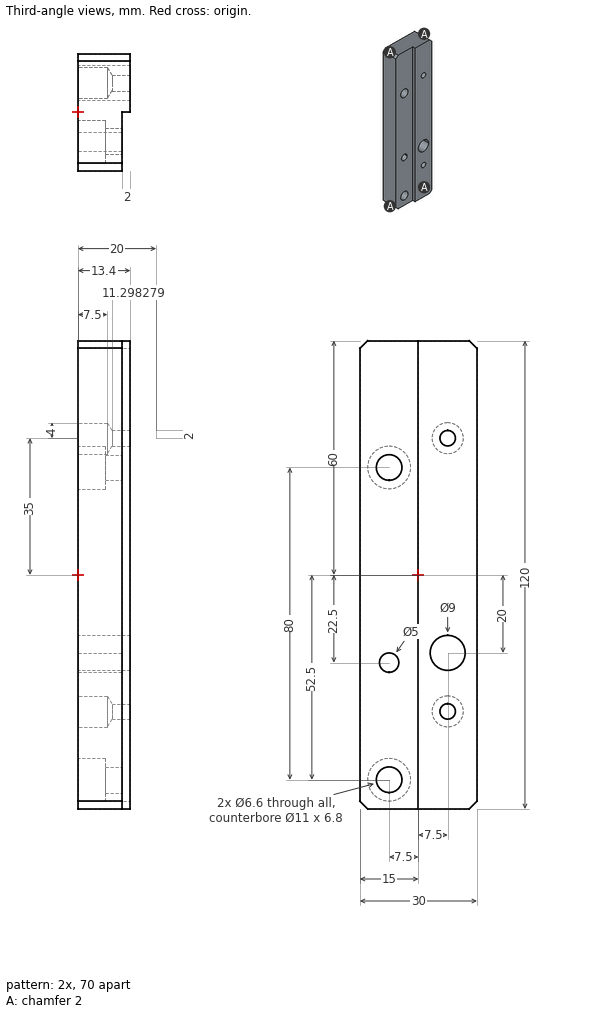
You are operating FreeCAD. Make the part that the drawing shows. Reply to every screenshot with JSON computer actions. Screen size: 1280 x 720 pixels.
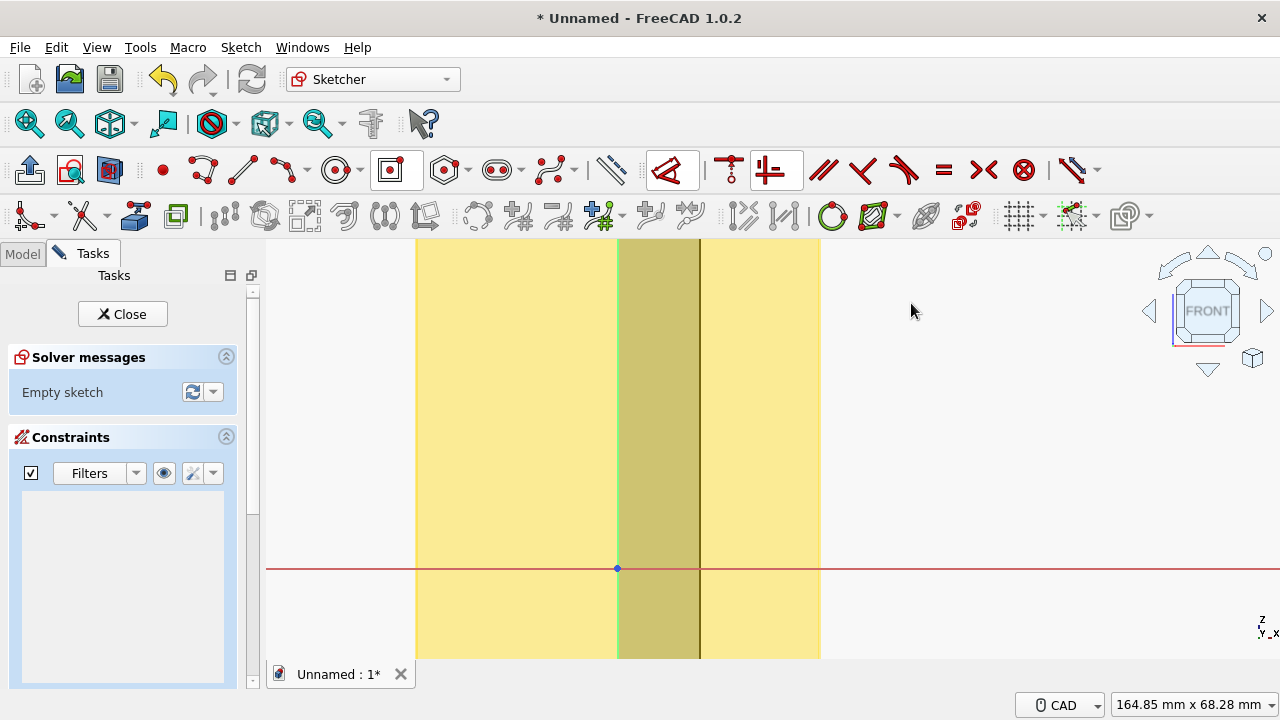
{"action": "left_click", "coordinate": [204, 170]}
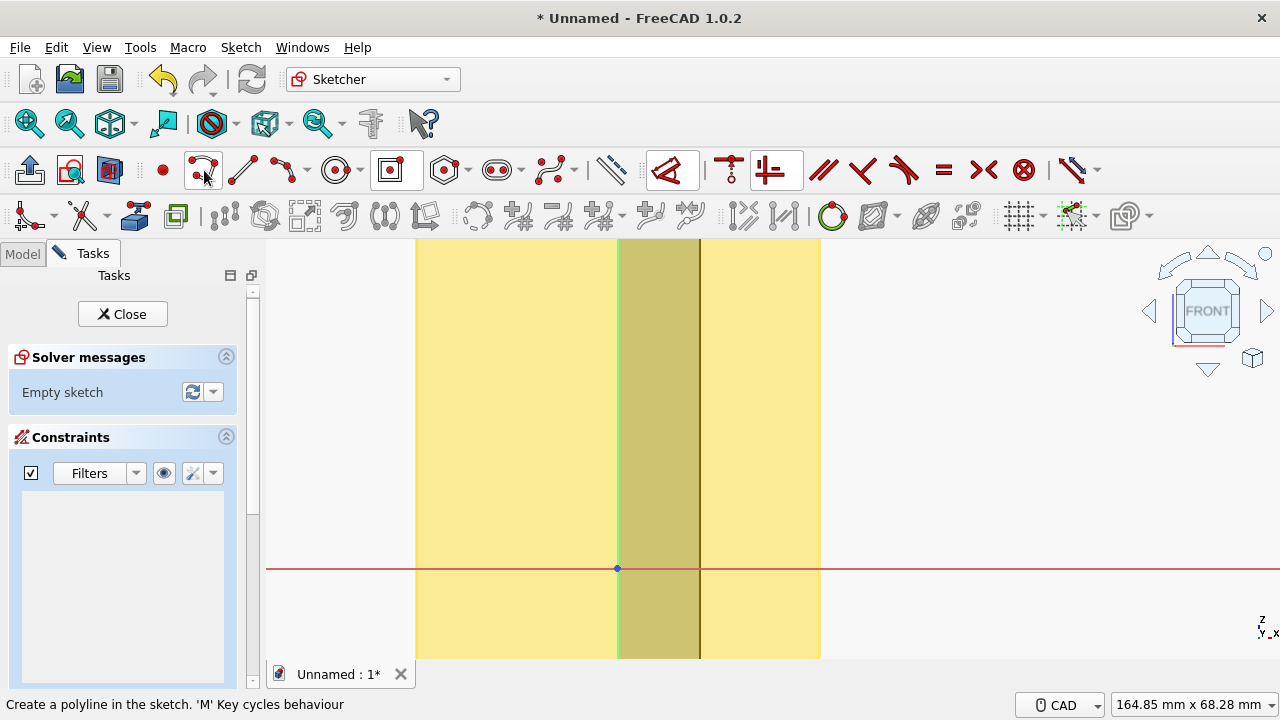
{"action": "left_click", "coordinate": [618, 354]}
{"action": "left_click", "coordinate": [627, 329]}
{"action": "left_click", "coordinate": [664, 329]}
{"action": "left_click", "coordinate": [671, 341]}
{"action": "left_click", "coordinate": [741, 341]}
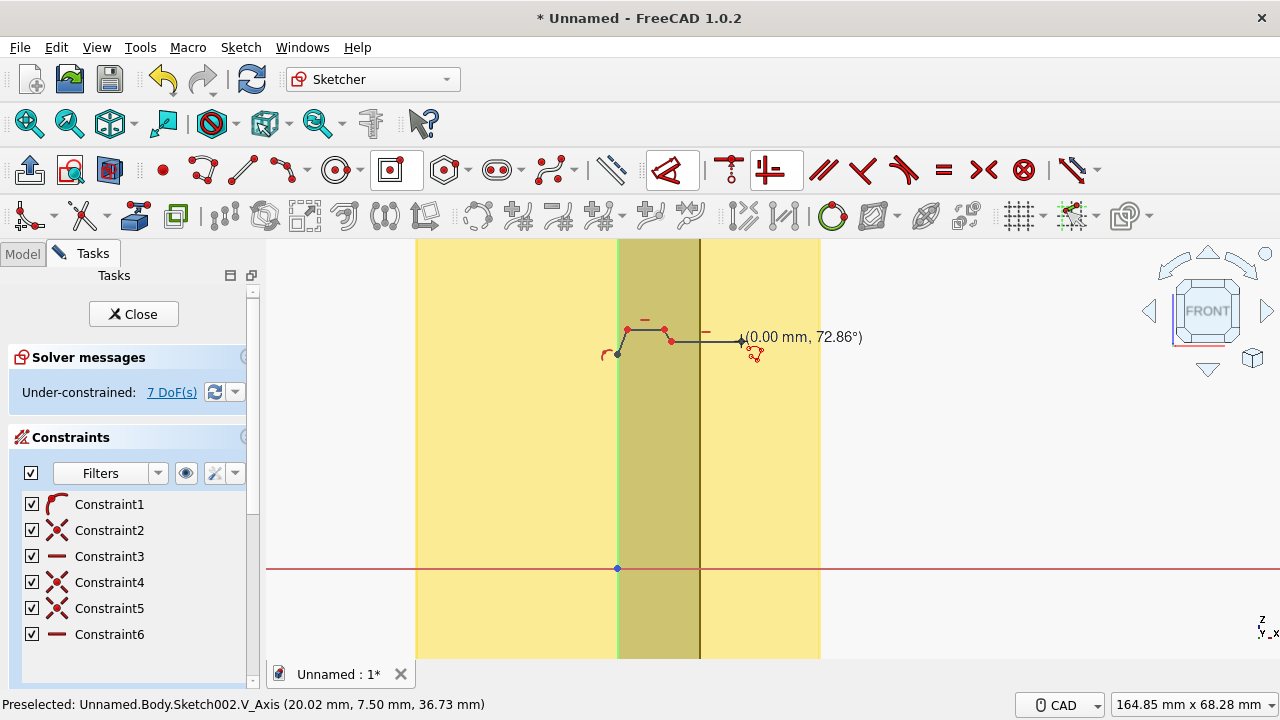
{"action": "scroll", "coordinate": [741, 354], "scroll_direction": "up", "scroll_amount": 2}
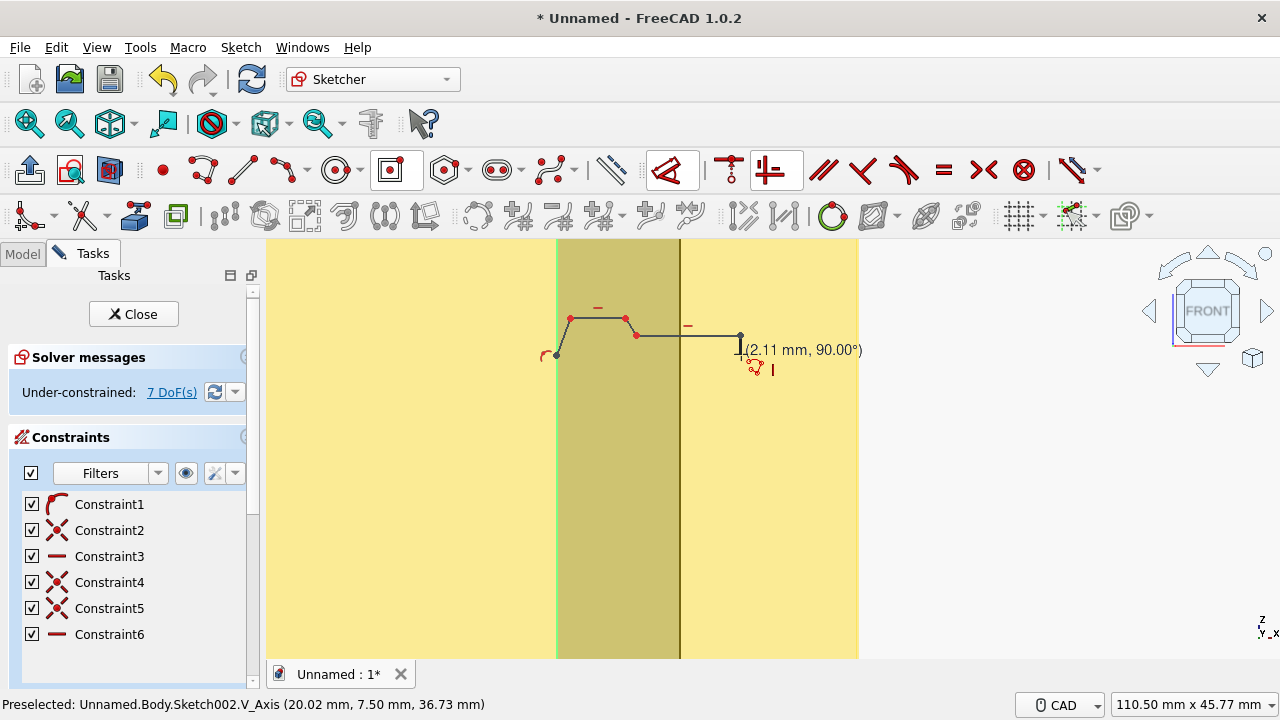
{"action": "left_click", "coordinate": [741, 353]}
{"action": "left_click", "coordinate": [557, 355]}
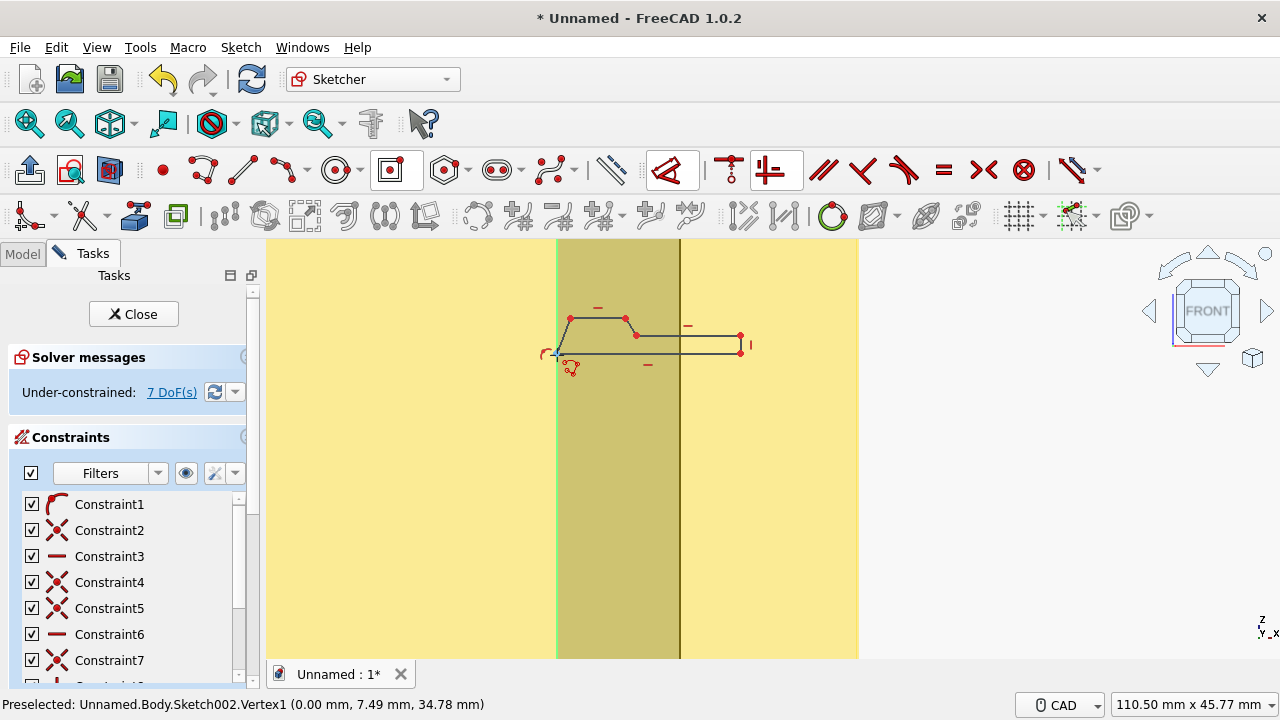
{"action": "left_click", "coordinate": [244, 170]}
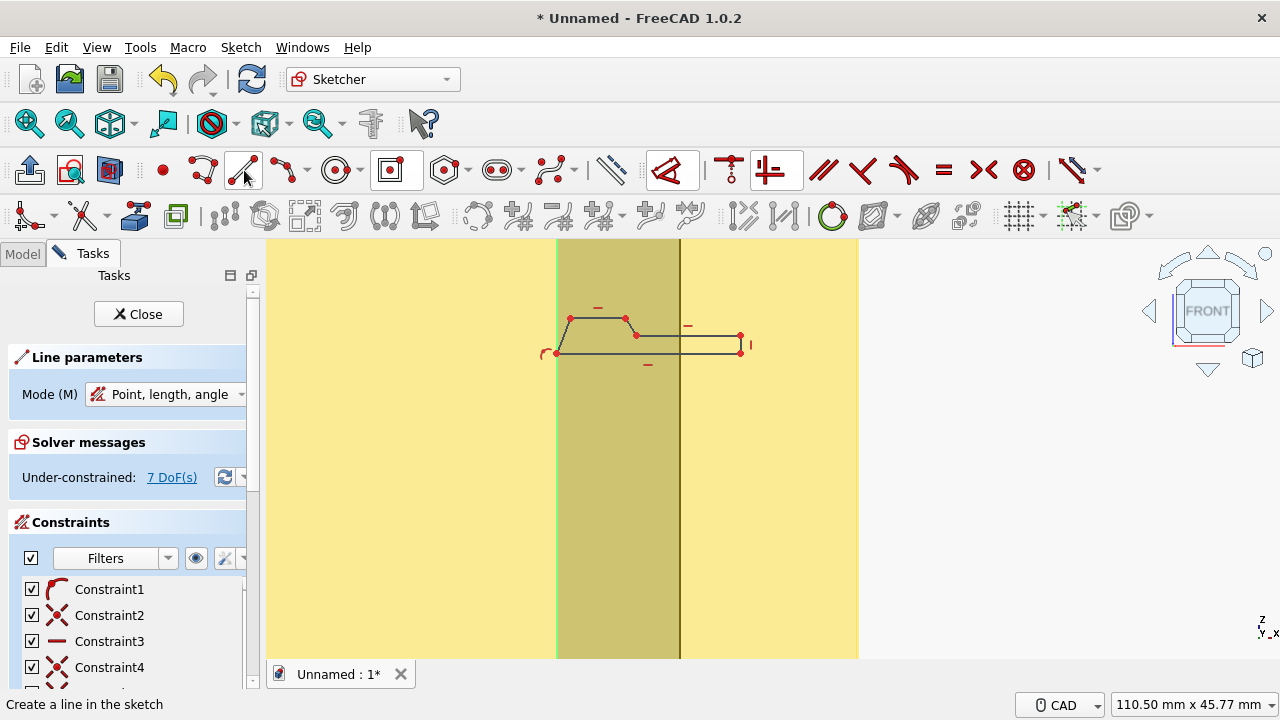
{"action": "left_click", "coordinate": [759, 353]}
{"action": "left_click", "coordinate": [814, 353]}
{"action": "key", "text": "Escape"}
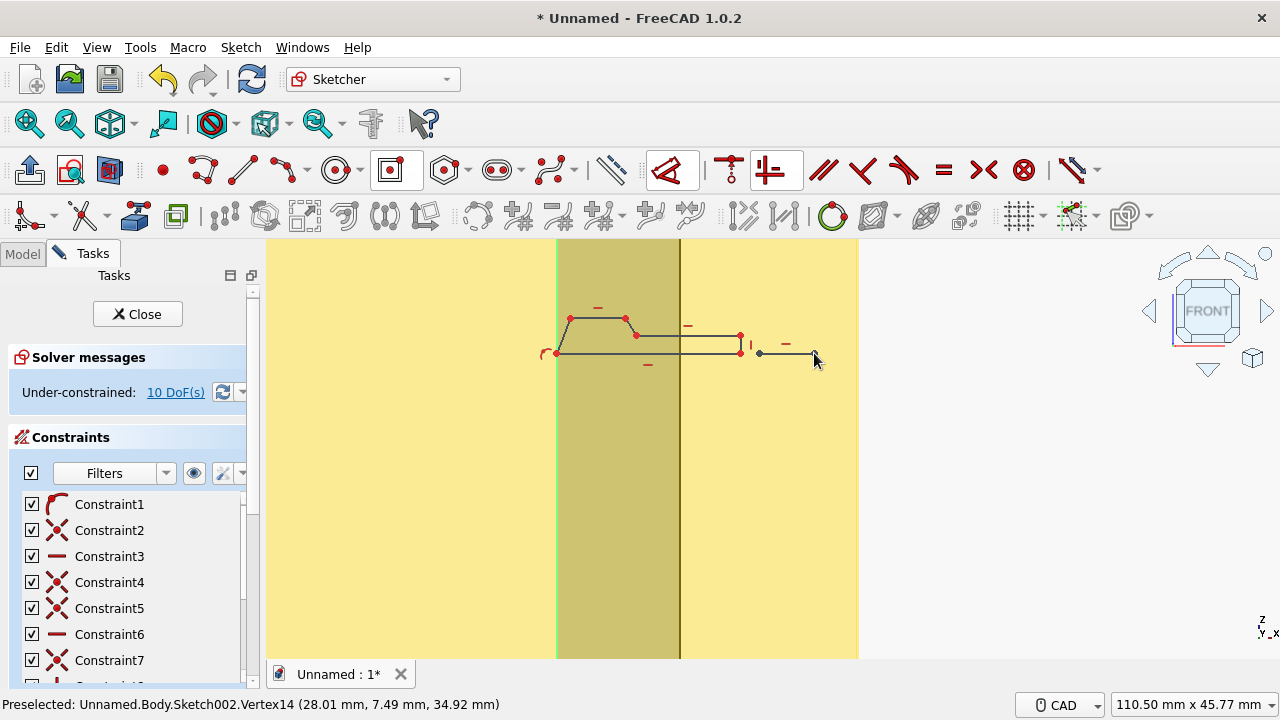
{"action": "left_click", "coordinate": [776, 354]}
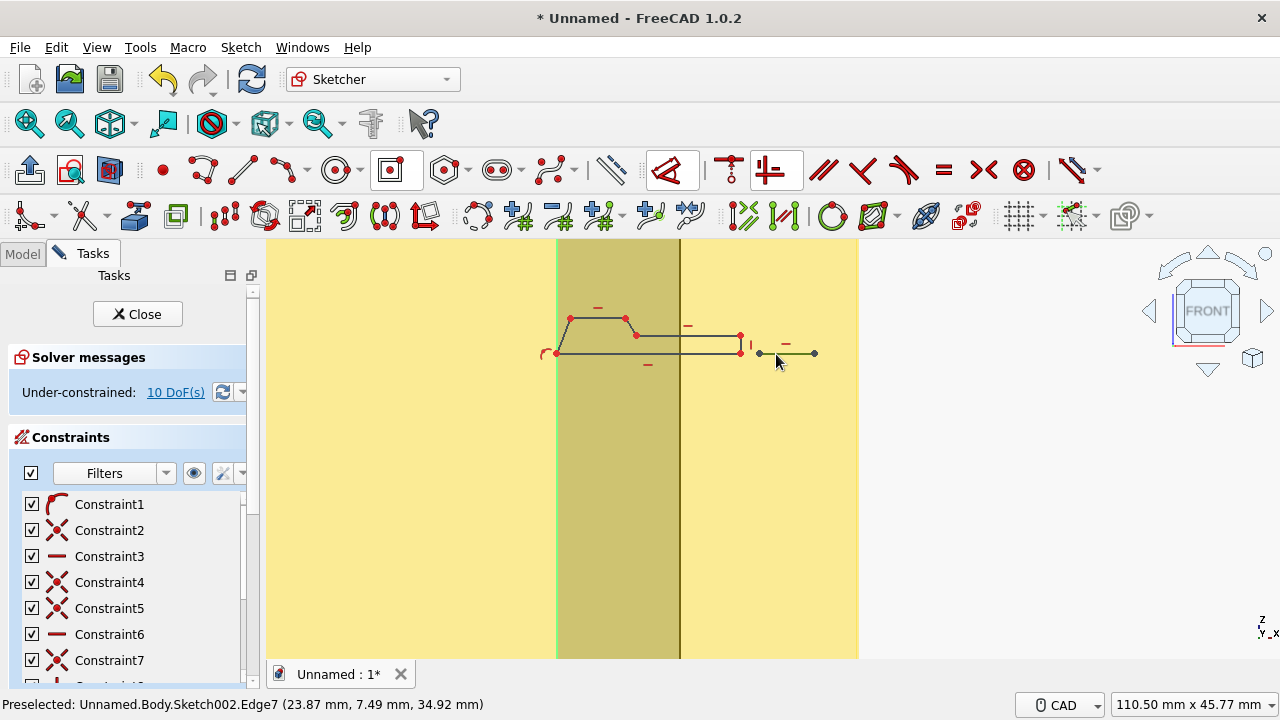
{"action": "left_click", "coordinate": [612, 170]}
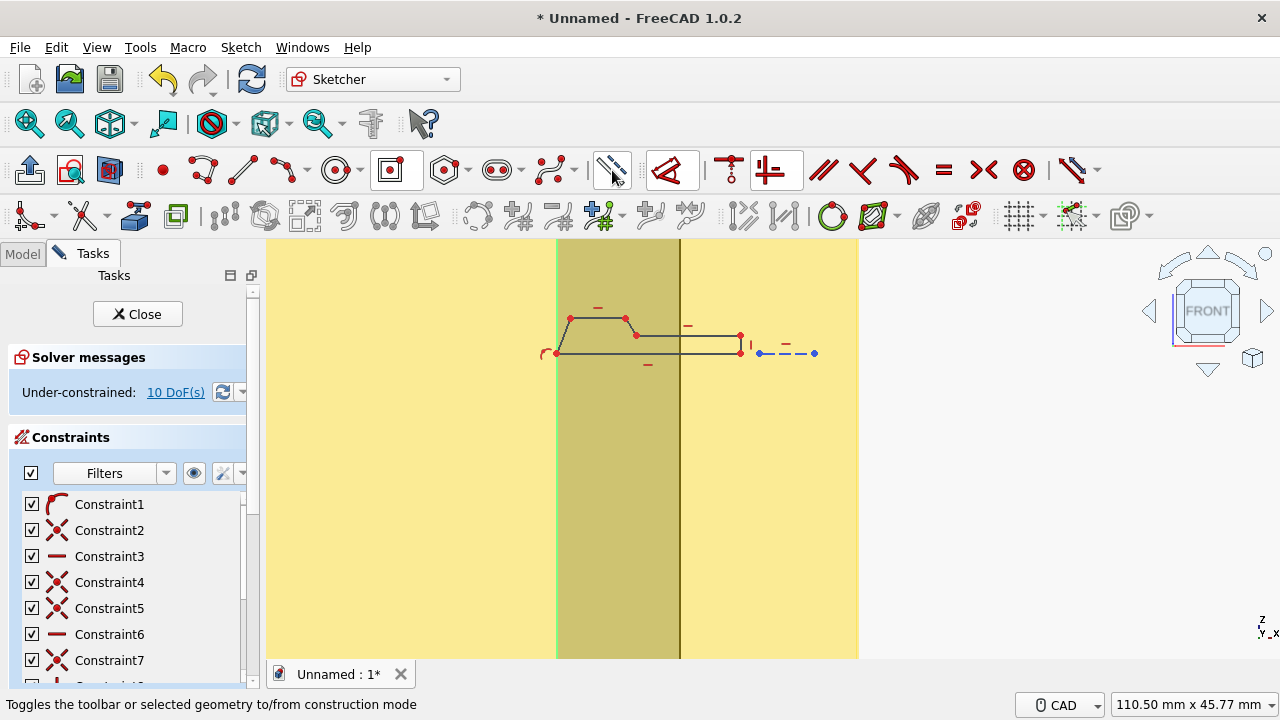
{"action": "scroll", "coordinate": [567, 329], "scroll_direction": "up", "scroll_amount": 2}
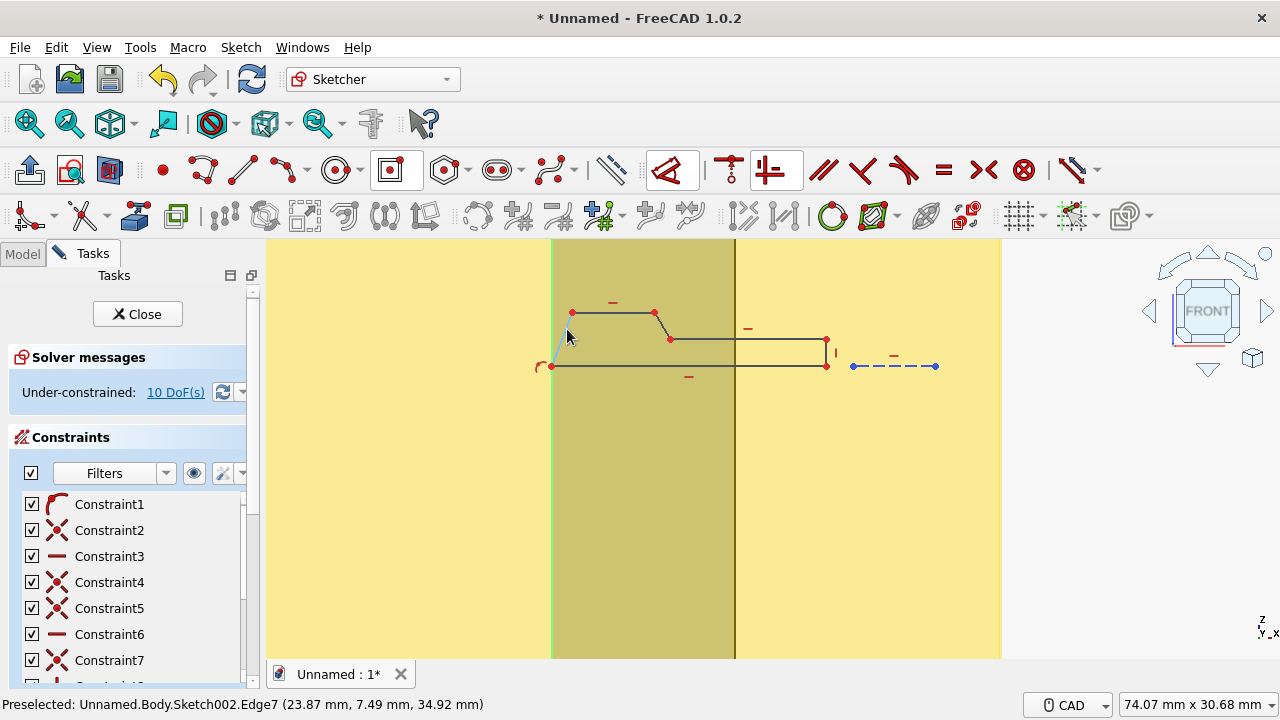
{"action": "left_click", "coordinate": [566, 329]}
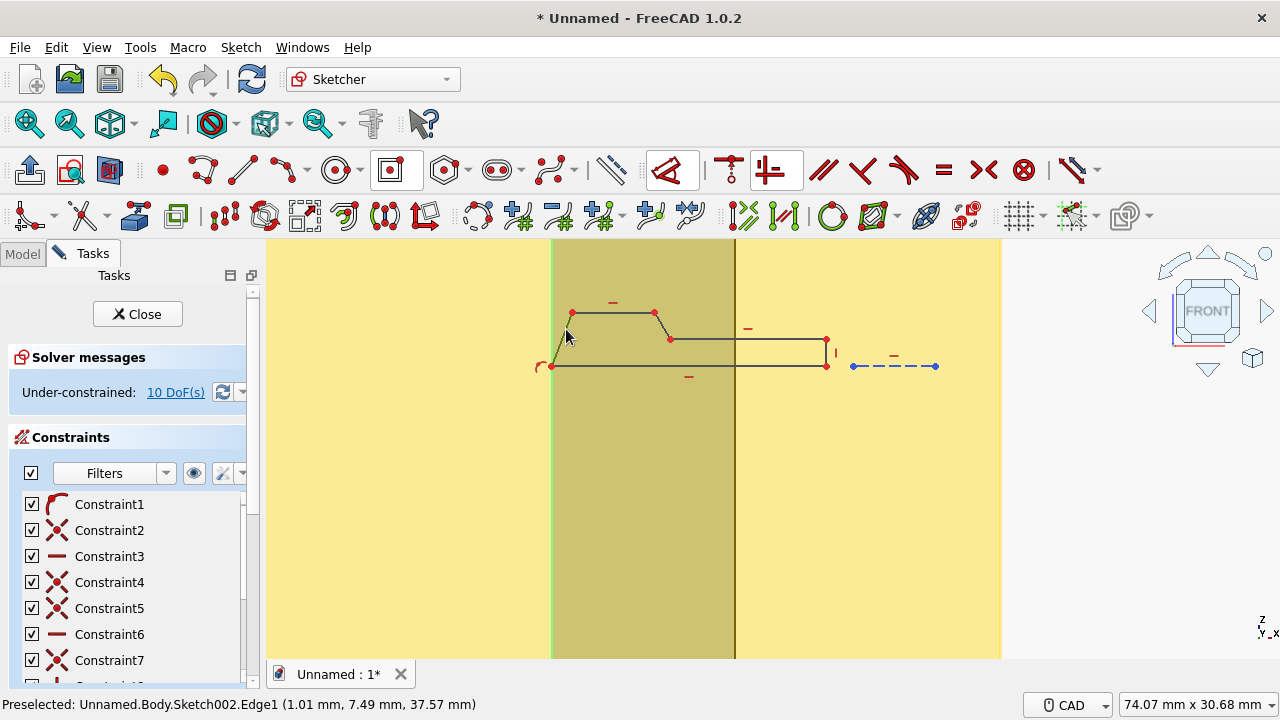
{"action": "key", "text": "v"}